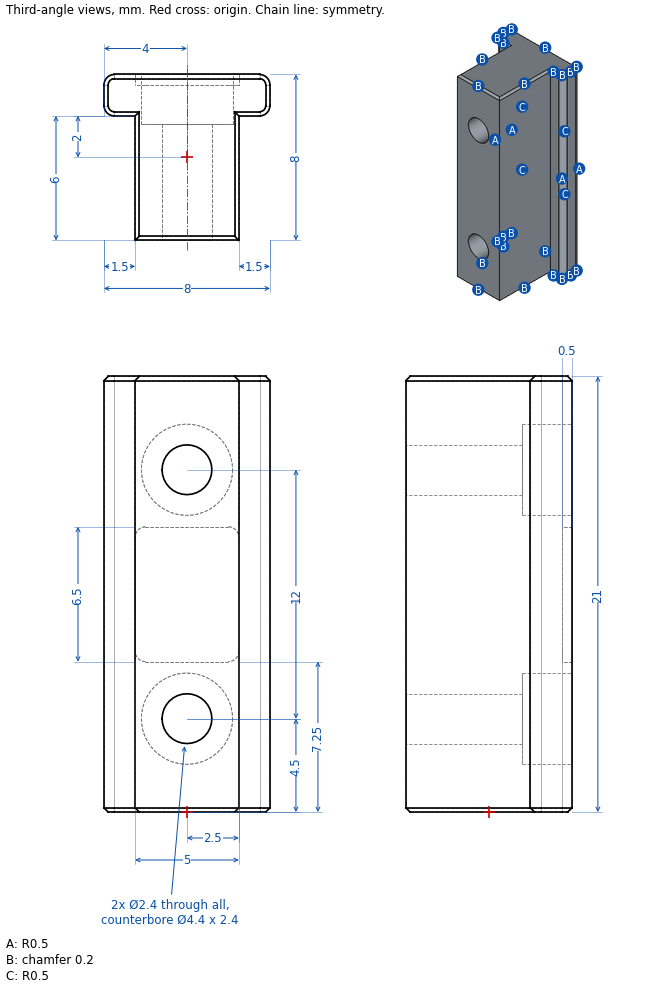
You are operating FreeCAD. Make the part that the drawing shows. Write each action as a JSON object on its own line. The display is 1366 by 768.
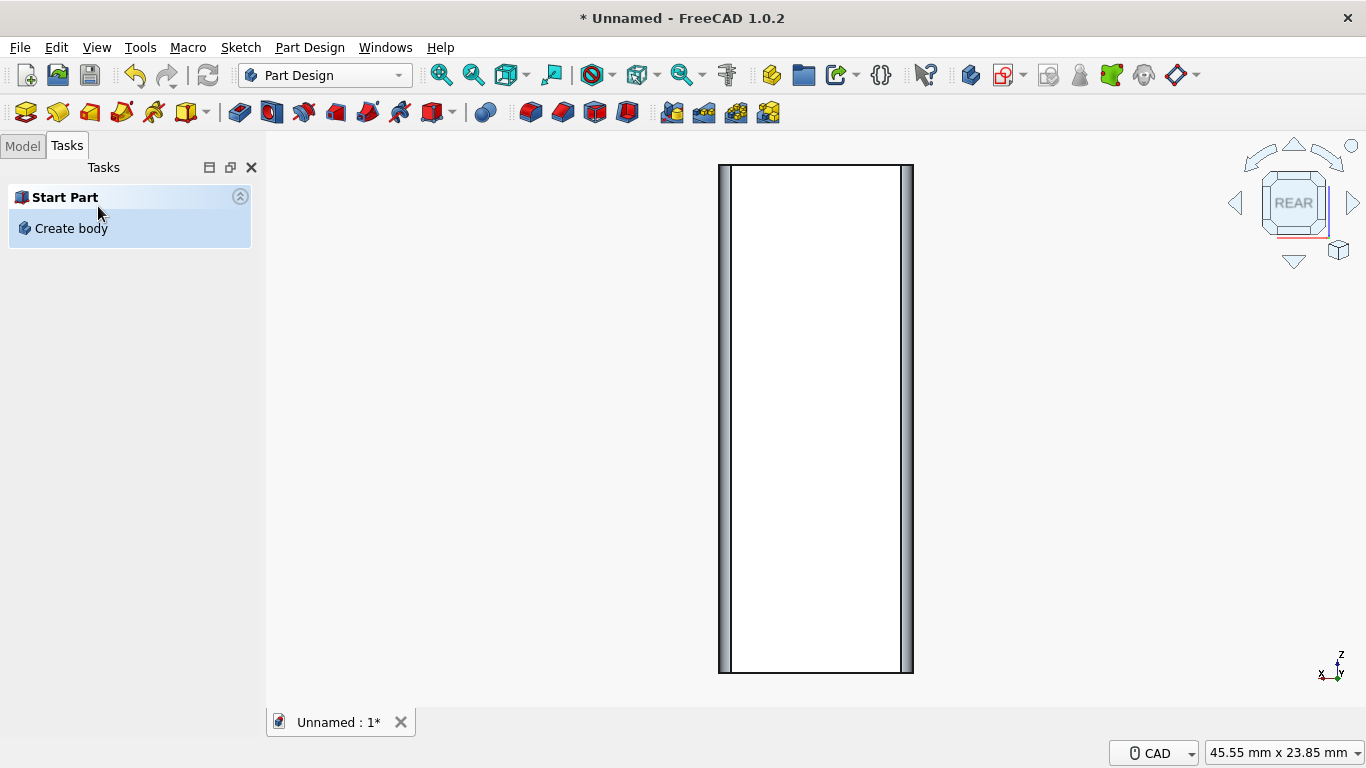
{"action": "left_click", "coordinate": [816, 273]}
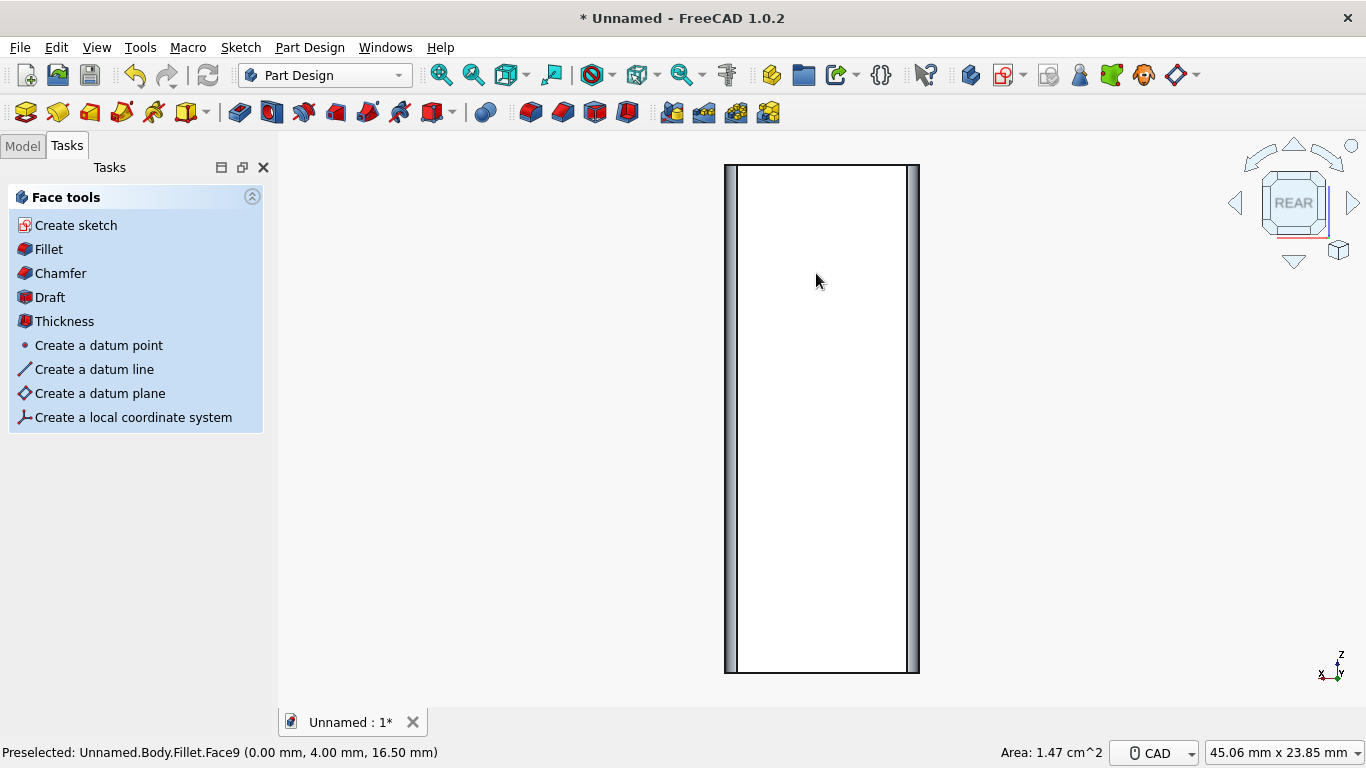
{"action": "left_click", "coordinate": [1004, 76]}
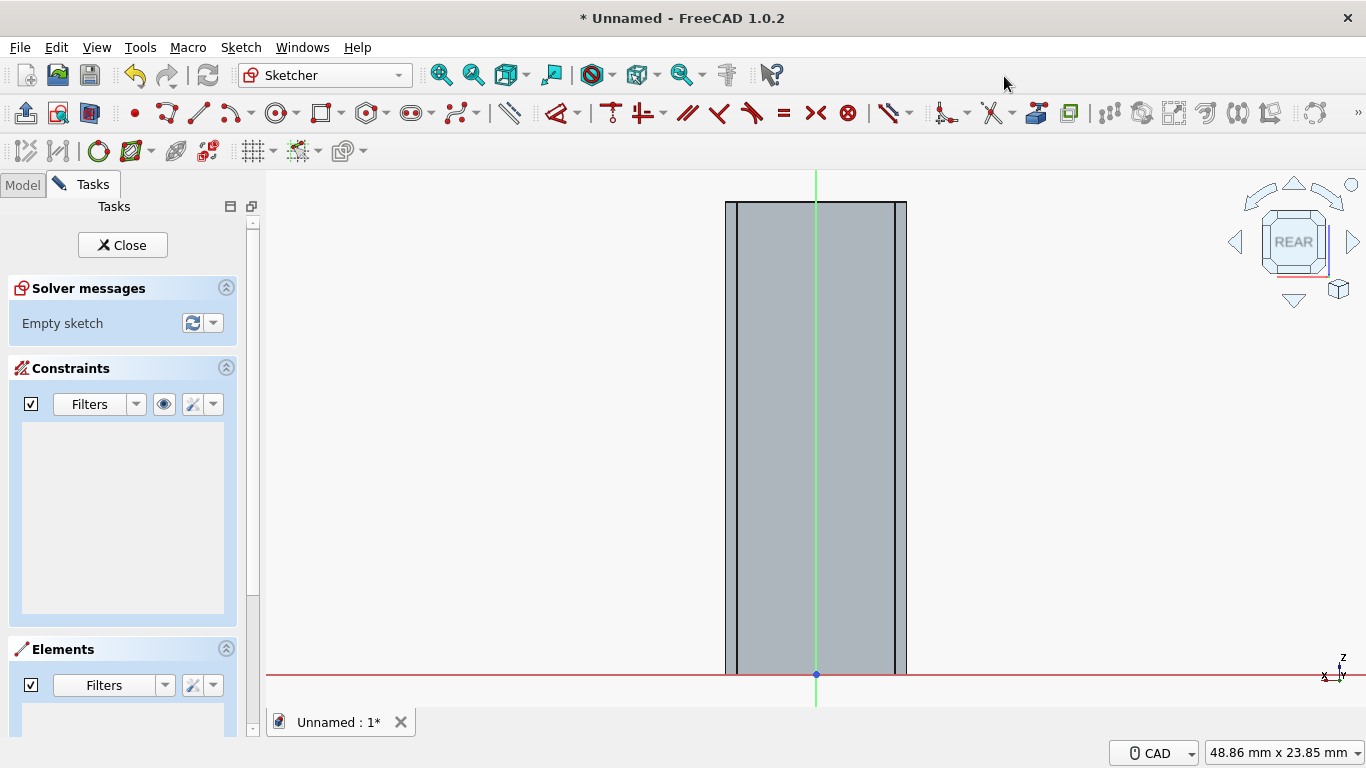
{"action": "scroll", "coordinate": [438, 271], "scroll_direction": "down", "scroll_amount": 1}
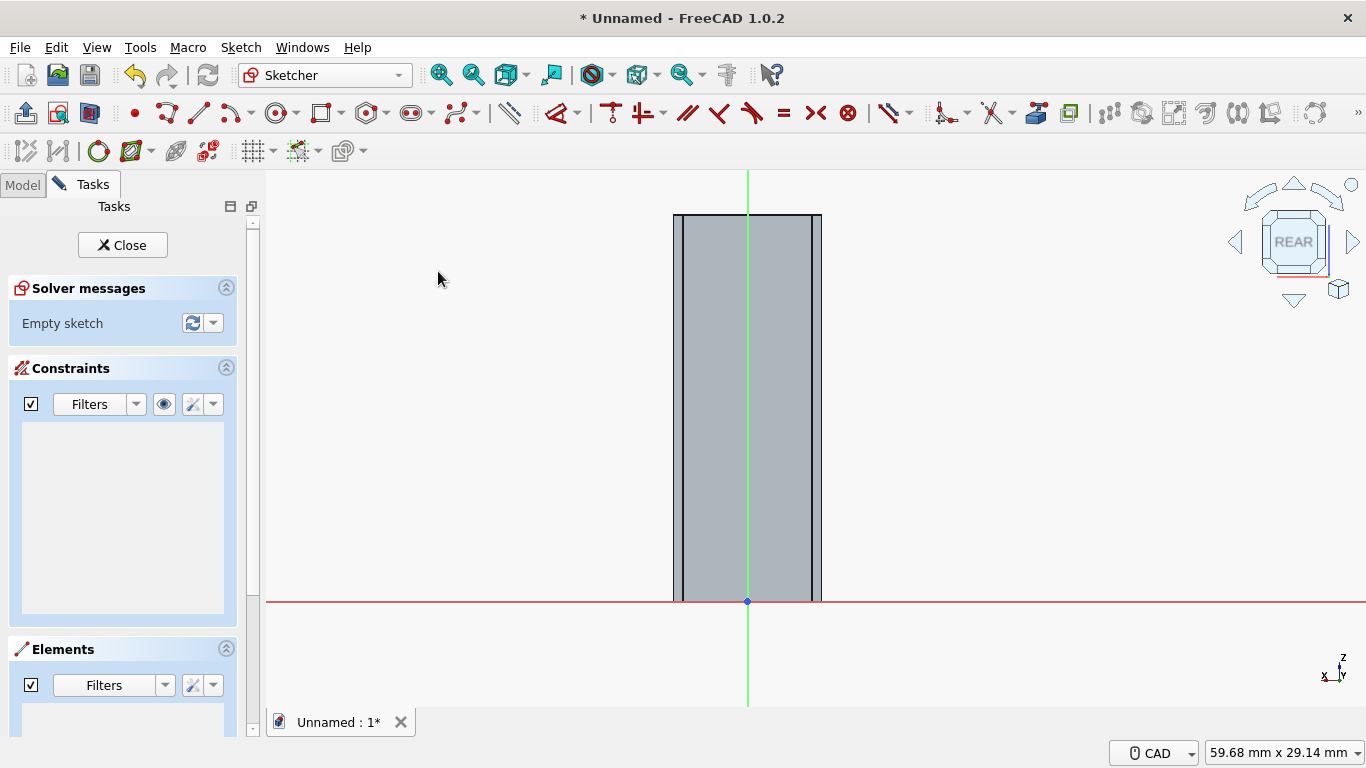
{"action": "left_click", "coordinate": [276, 114]}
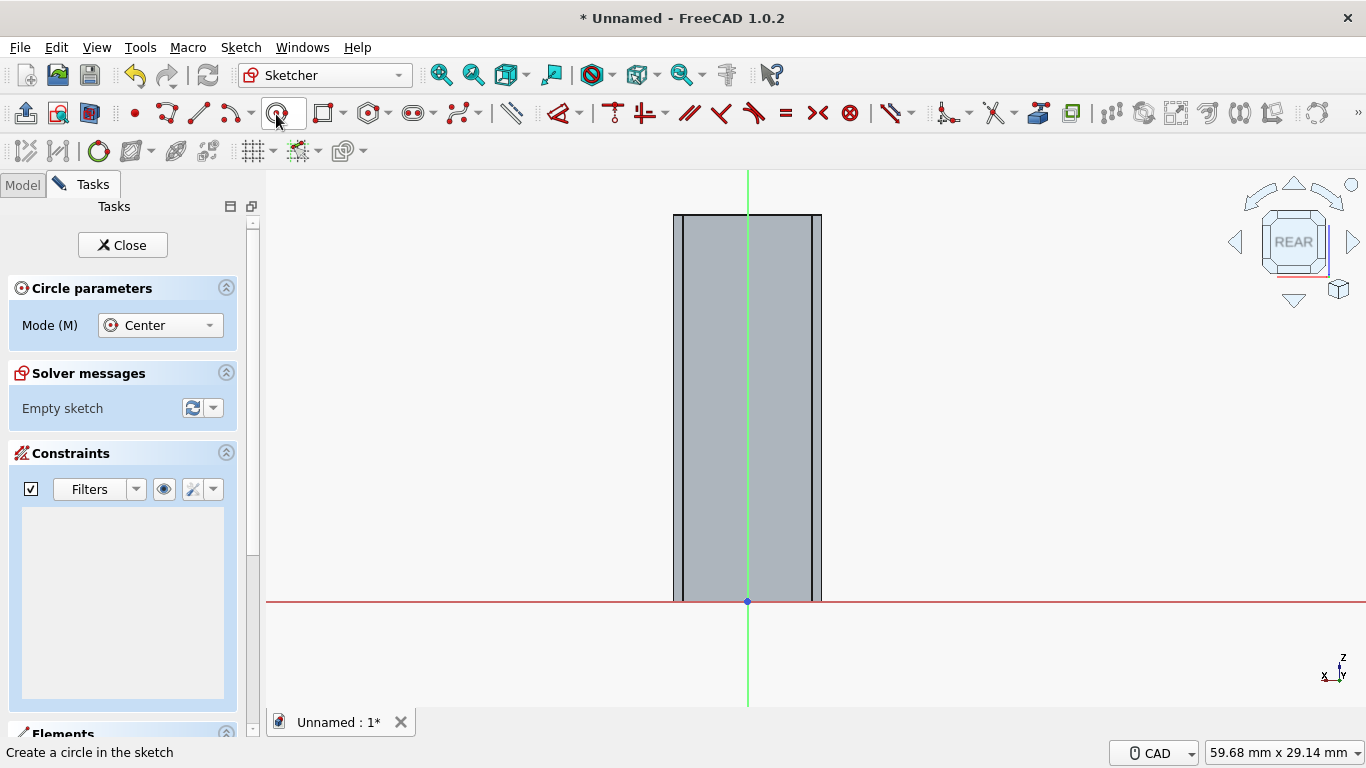
{"action": "left_click", "coordinate": [748, 519]}
{"action": "mouse_move", "coordinate": [763, 503]}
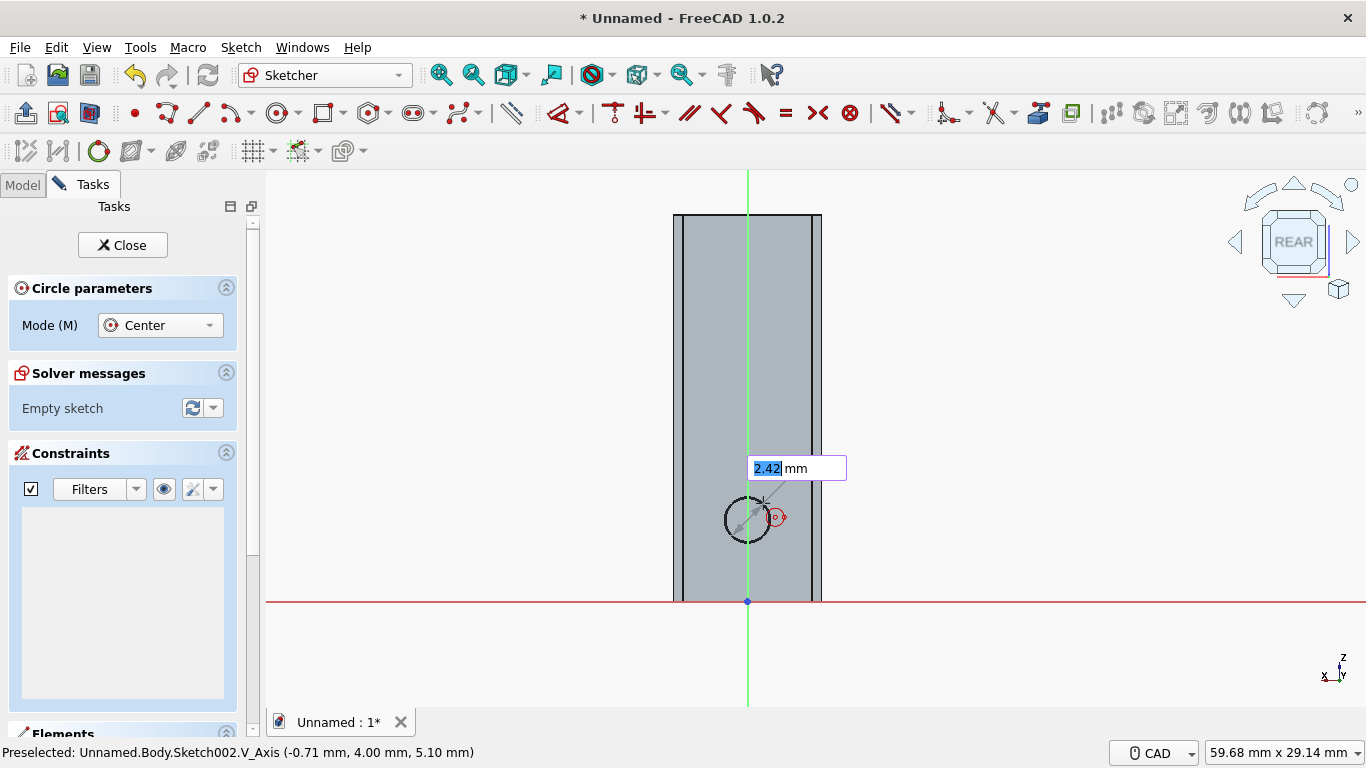
{"action": "type", "text": "2.4"}
{"action": "key", "text": "Return"}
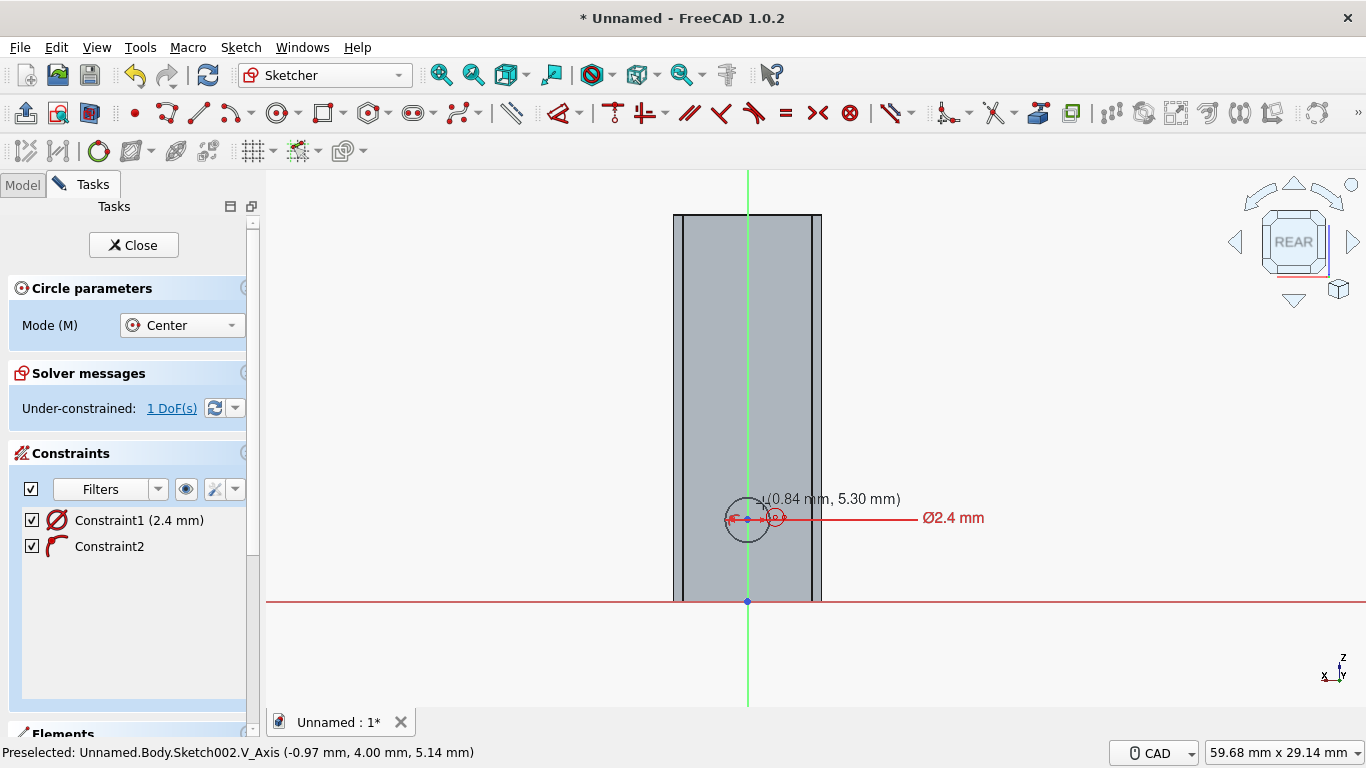
{"action": "left_click", "coordinate": [748, 298]}
{"action": "mouse_move", "coordinate": [763, 282]}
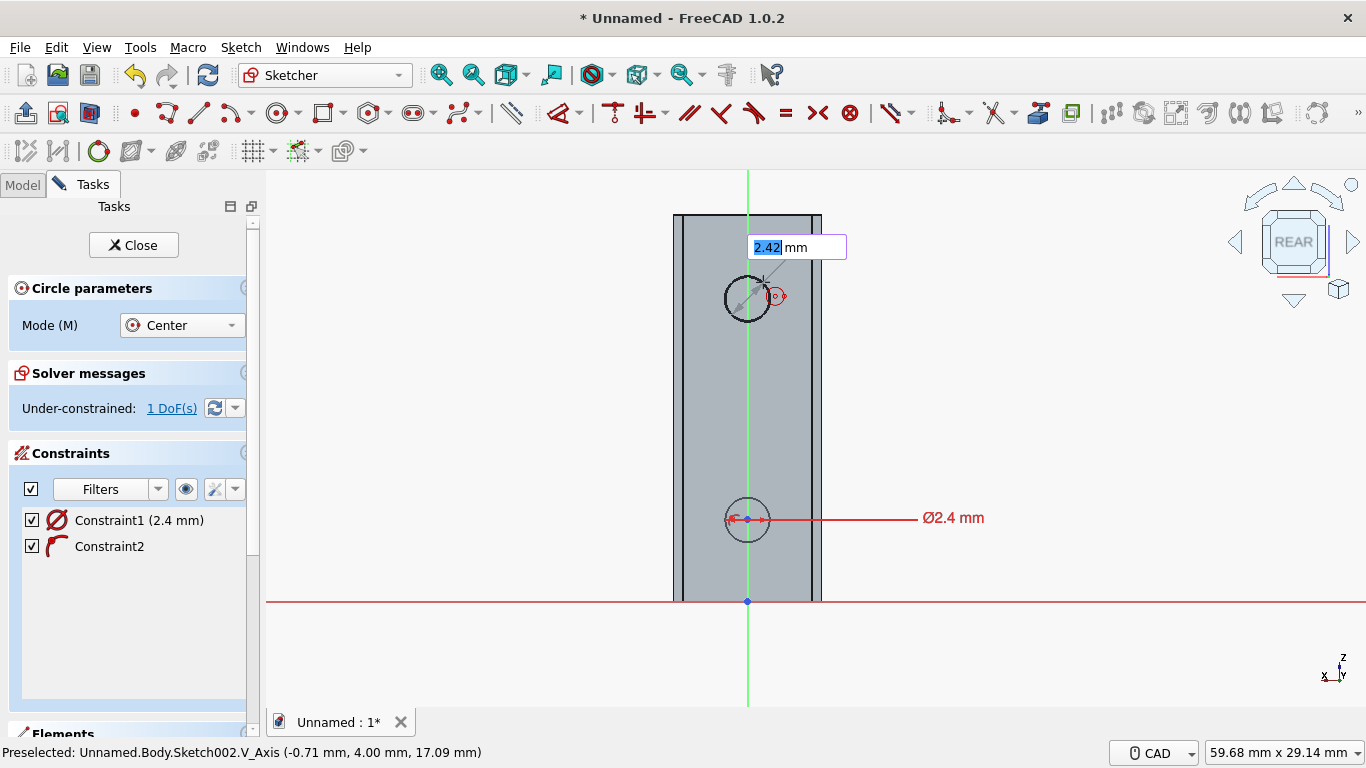
{"action": "type", "text": "2.4"}
{"action": "key", "text": "Return"}
{"action": "key", "text": "Escape"}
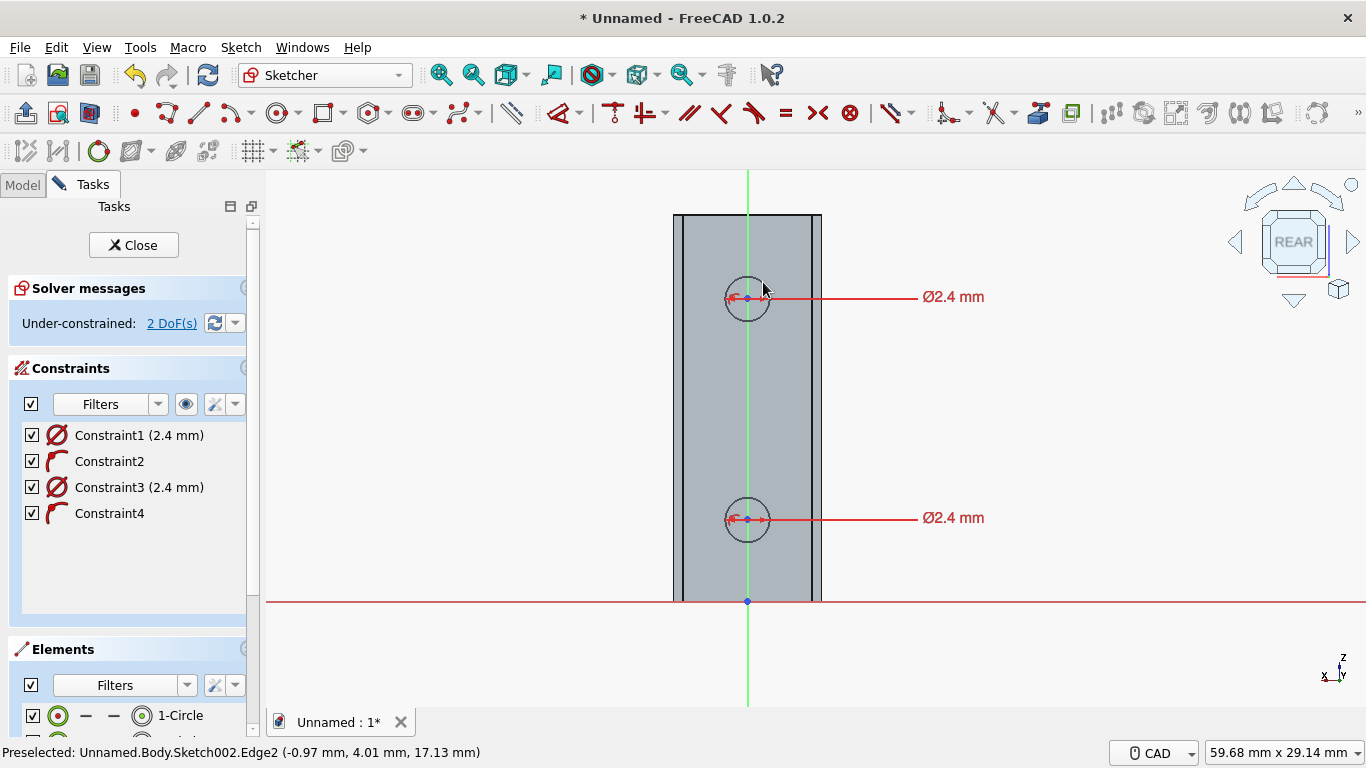
{"action": "left_click", "coordinate": [558, 114]}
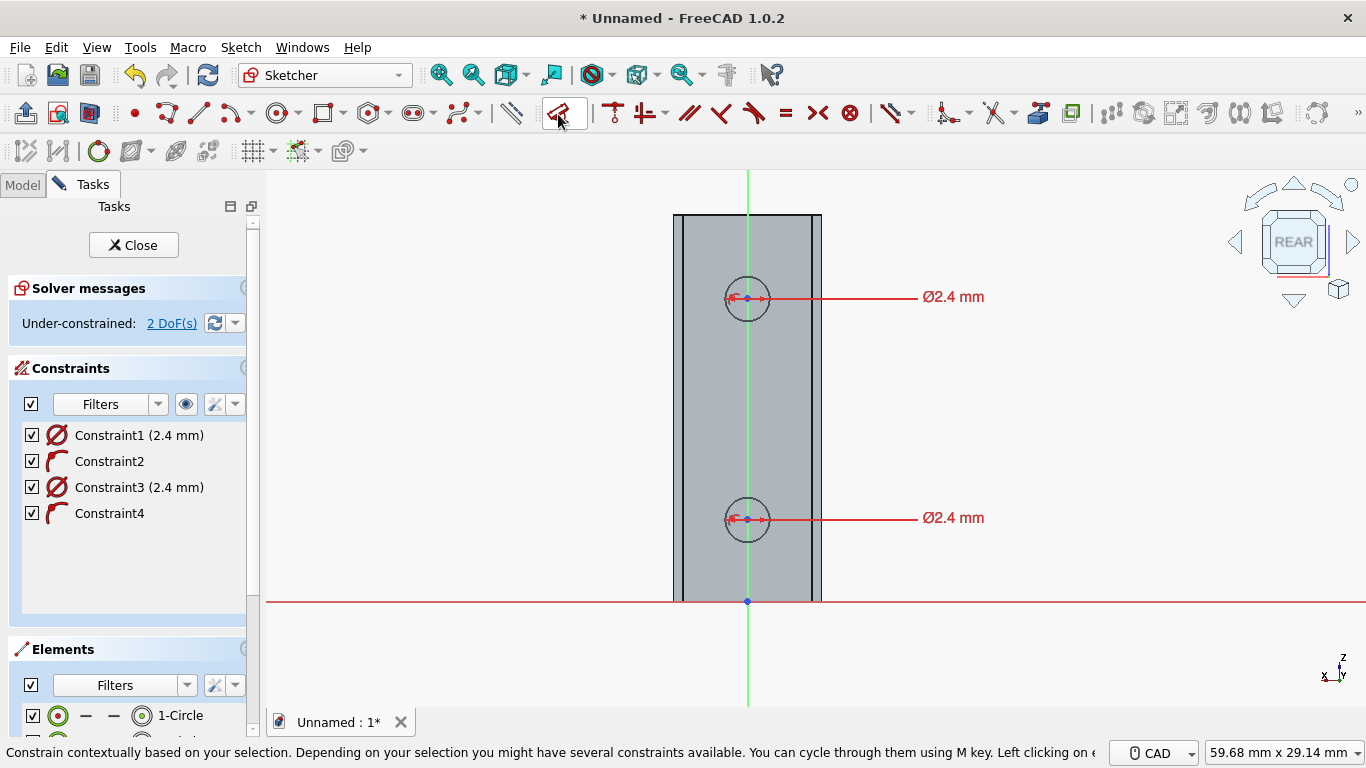
{"action": "left_click", "coordinate": [748, 520]}
{"action": "left_click", "coordinate": [782, 561]}